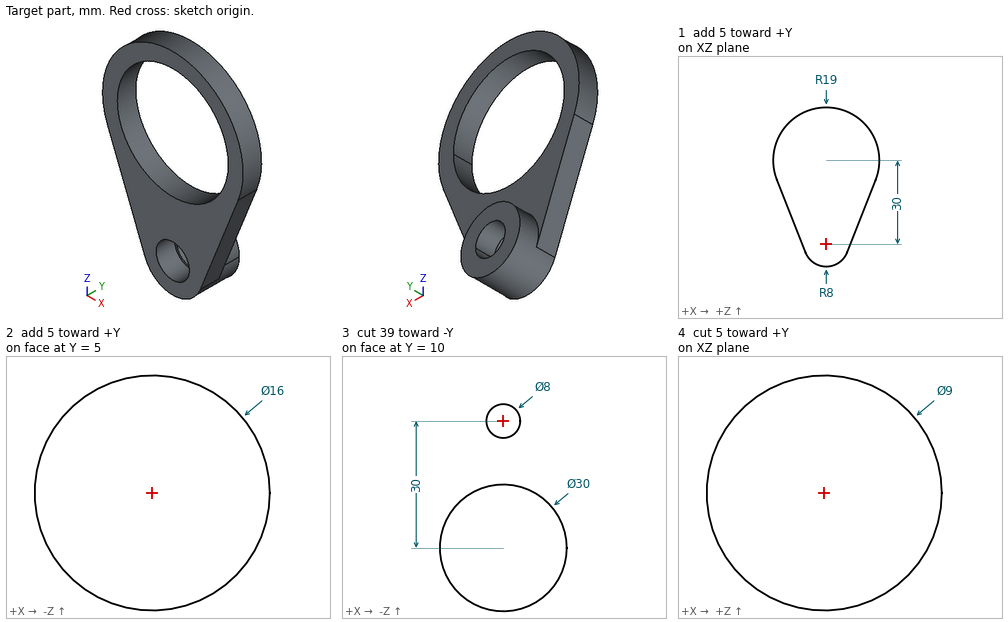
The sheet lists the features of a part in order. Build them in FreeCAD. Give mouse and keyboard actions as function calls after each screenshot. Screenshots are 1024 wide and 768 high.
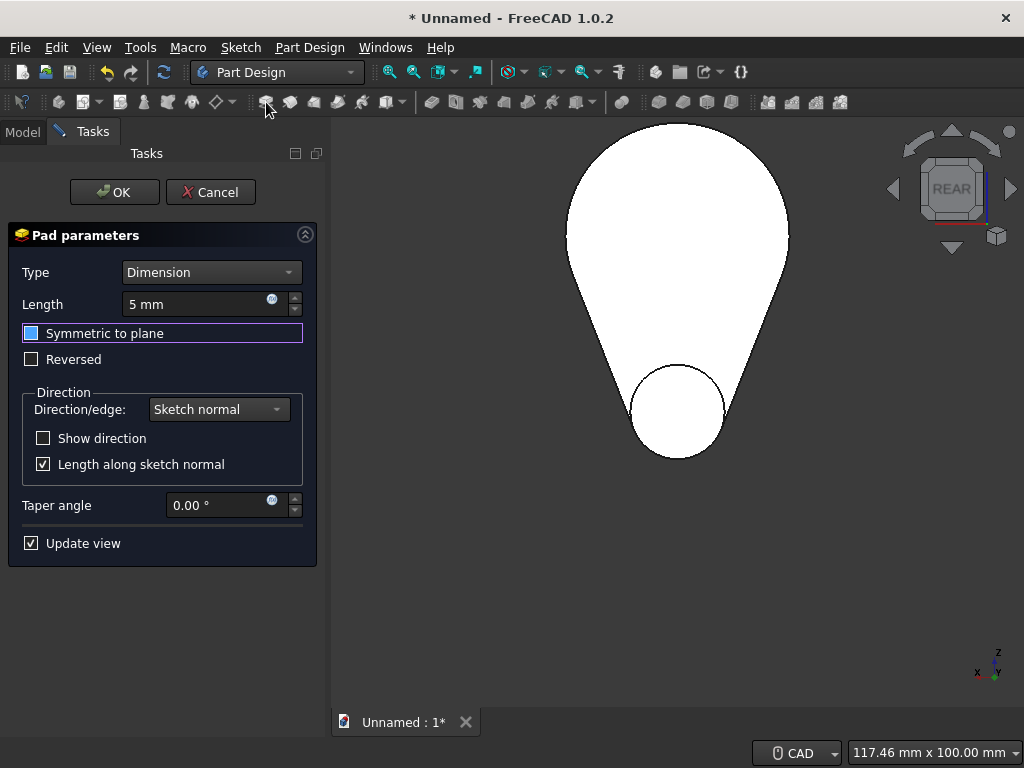
click(115, 192)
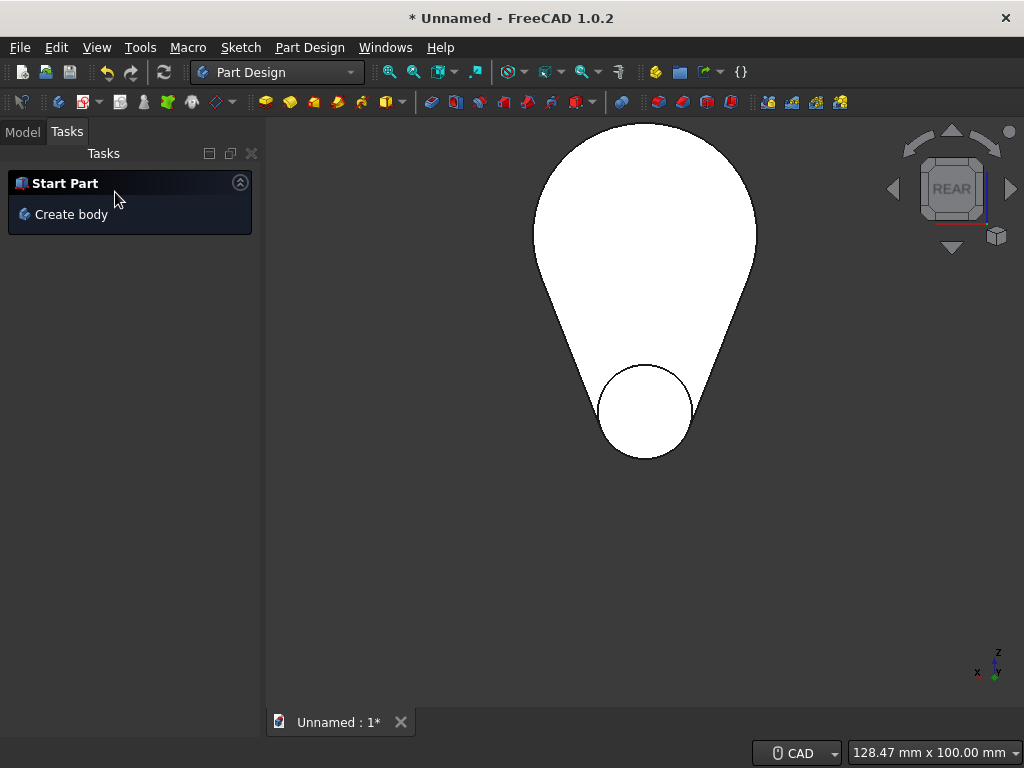
click(645, 411)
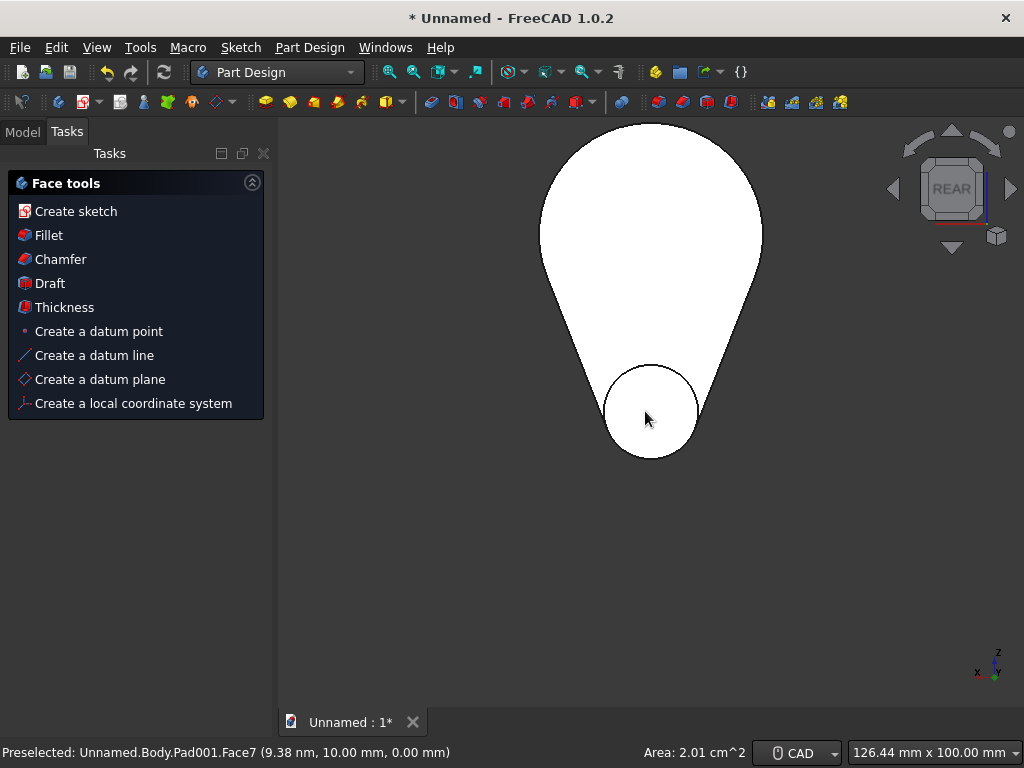
click(84, 102)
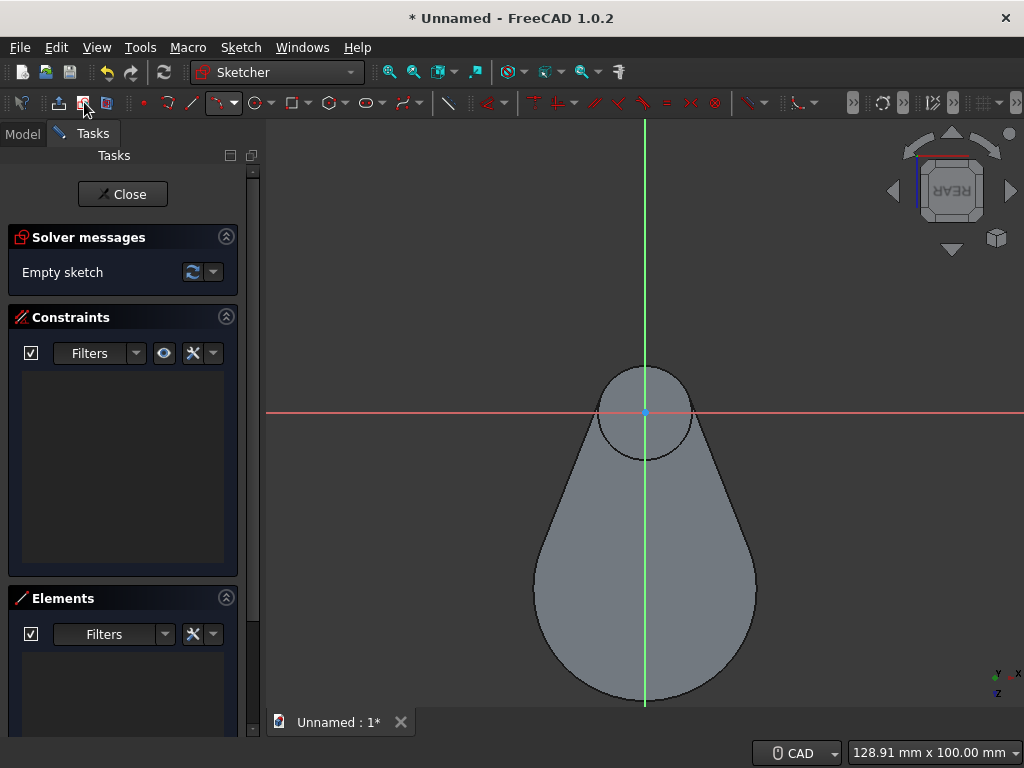
scroll(294, 147, down, 1)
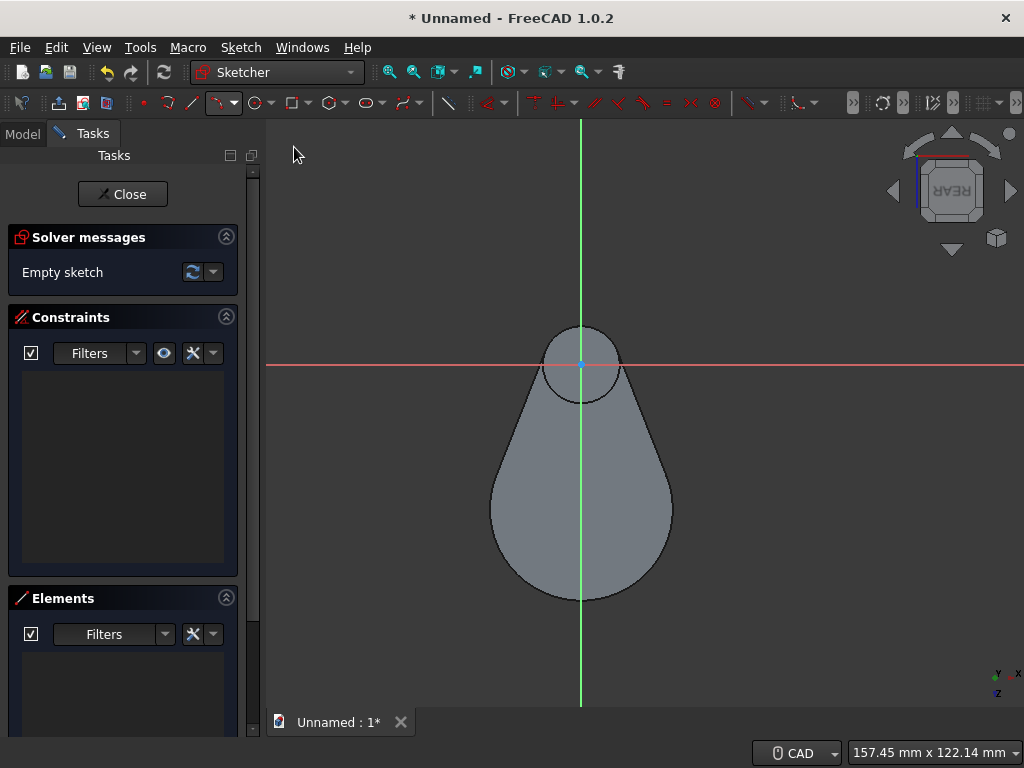
scroll(591, 566, up, 2)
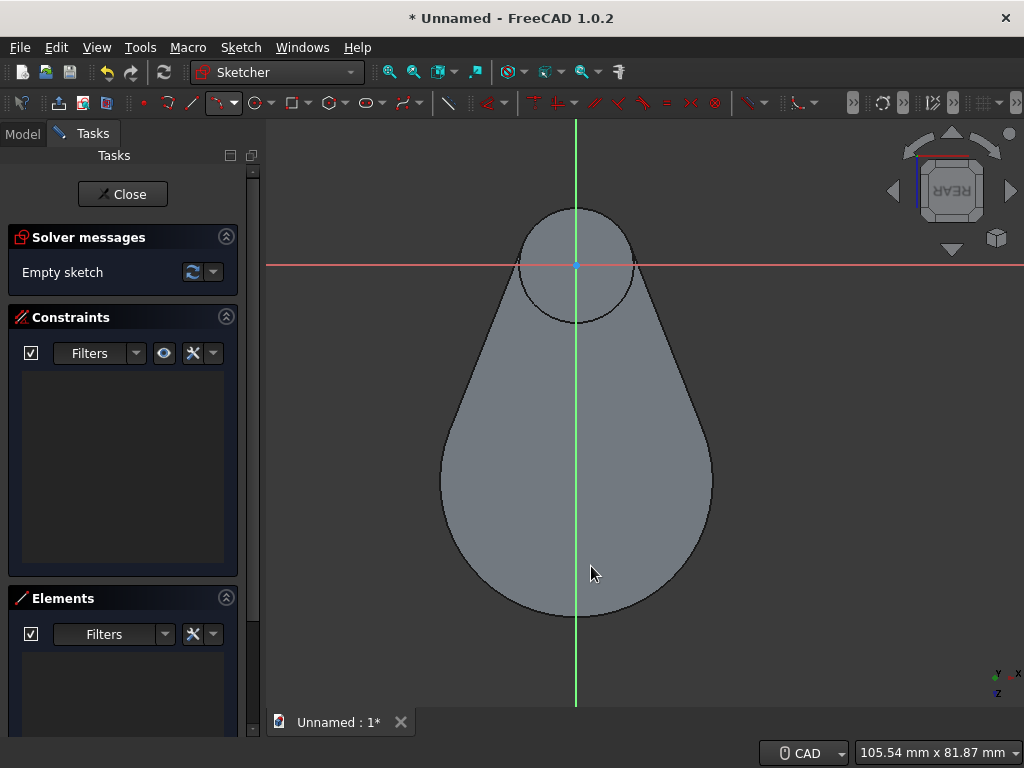
click(256, 104)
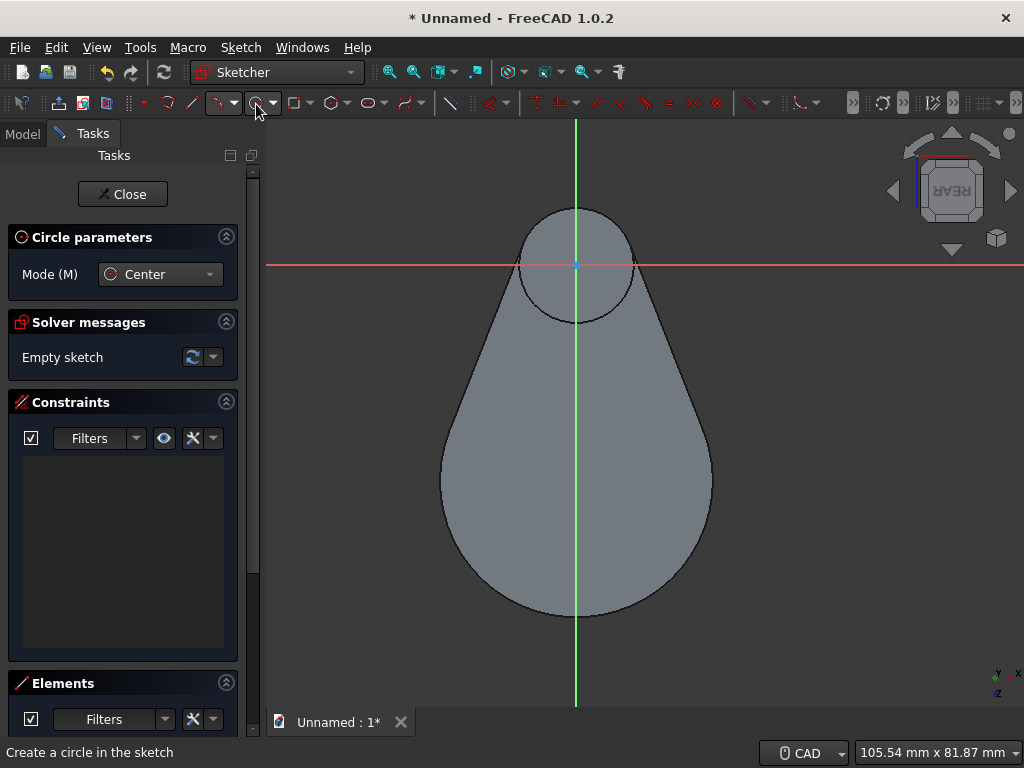
click(576, 265)
move(597, 245)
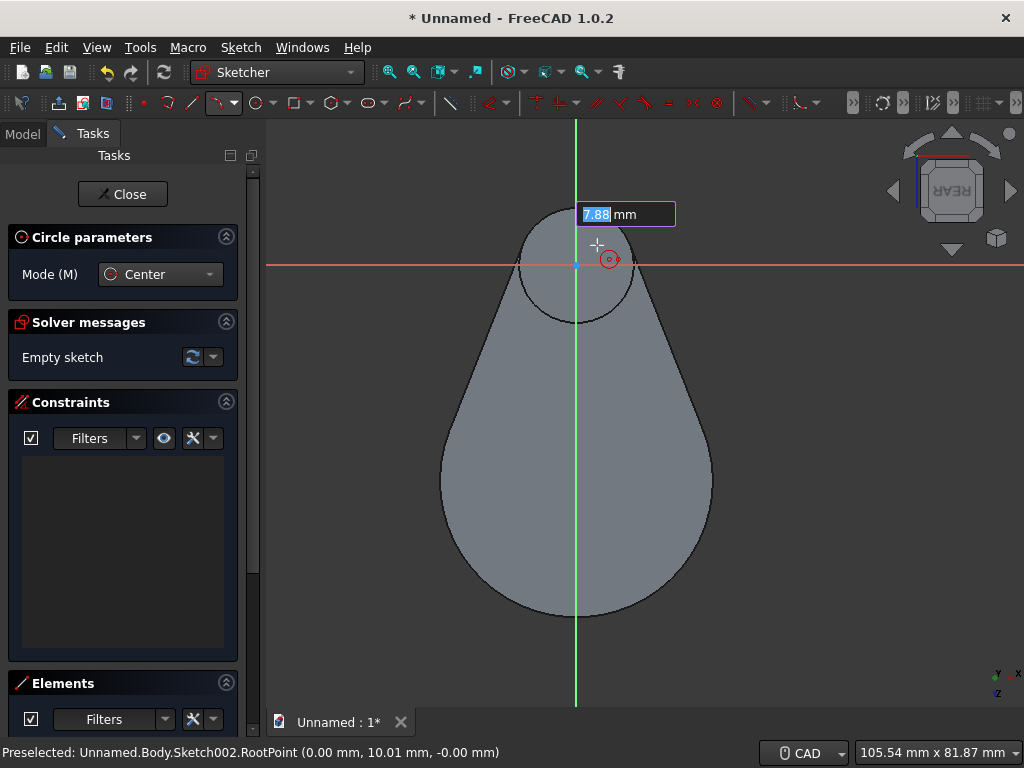
text(8)
key(Return)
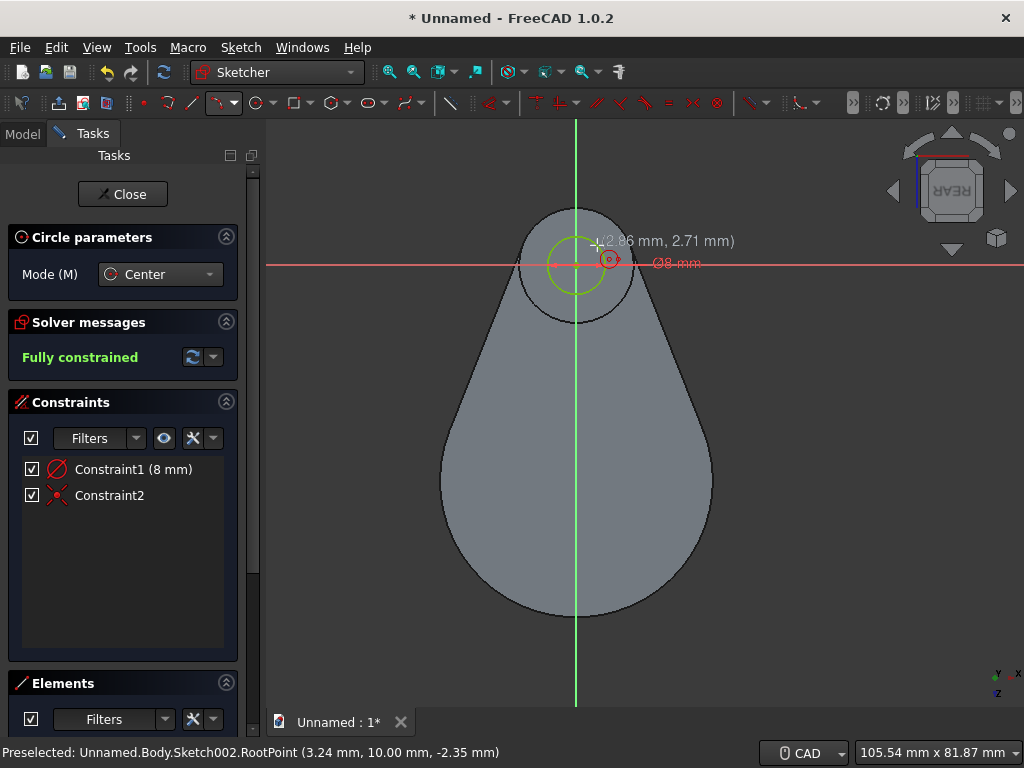
click(576, 481)
move(653, 405)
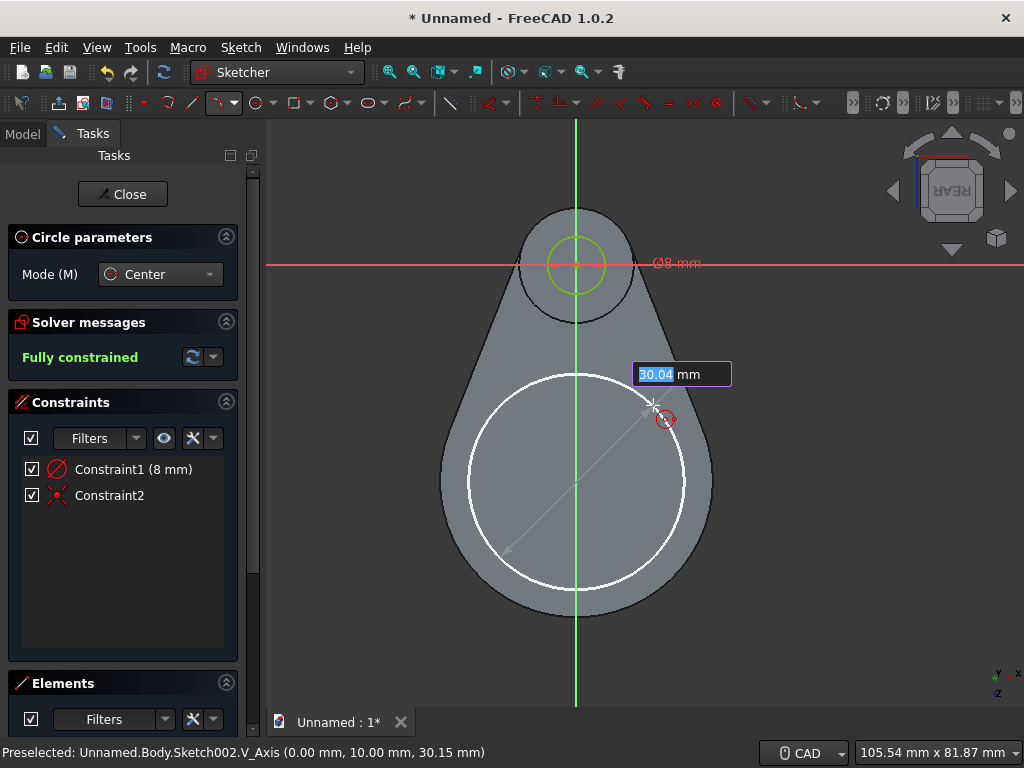
text(30)
key(Return)
key(Escape)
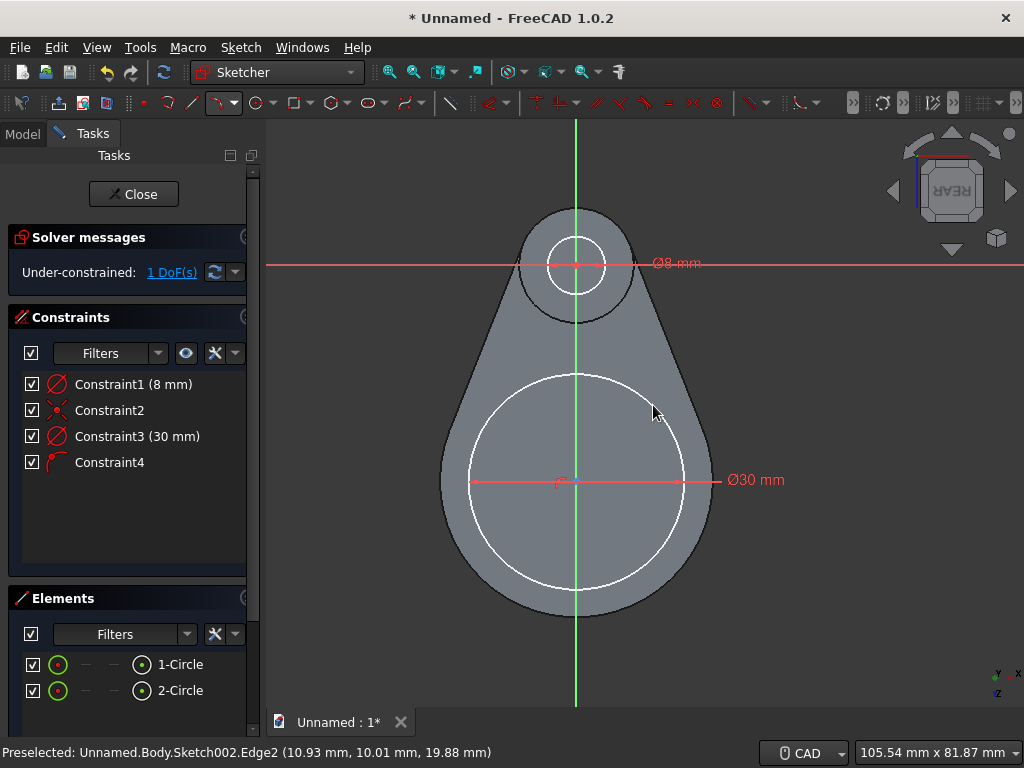
click(490, 104)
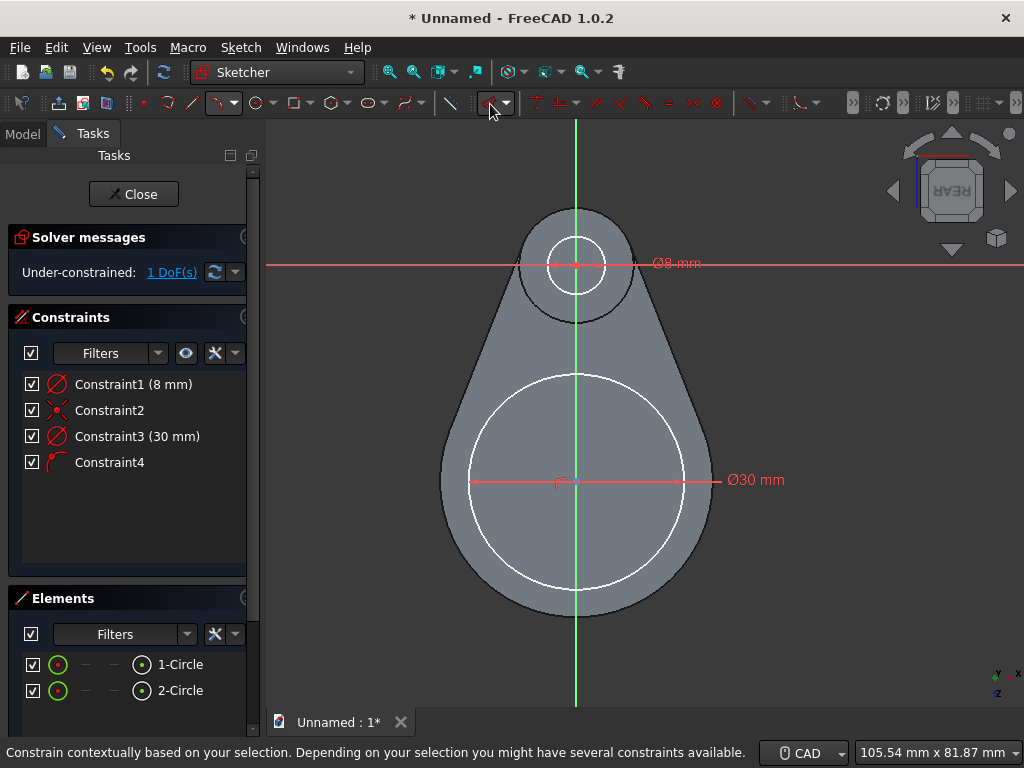
click(576, 482)
click(610, 324)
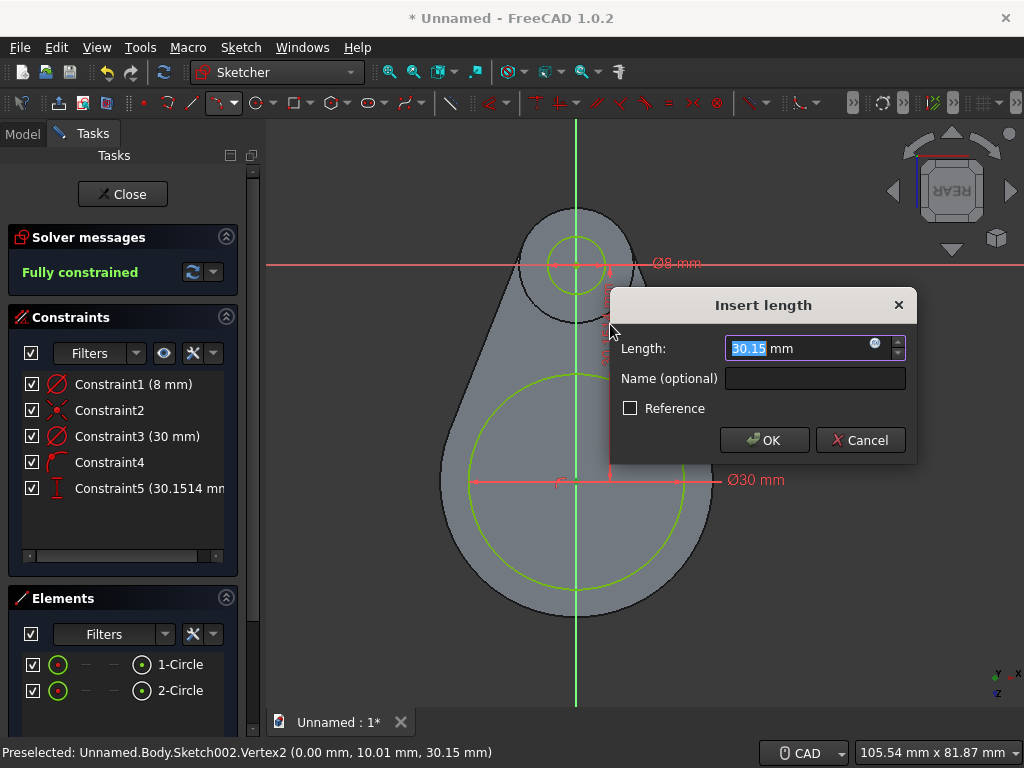
text(30)
key(Return)
key(Escape)